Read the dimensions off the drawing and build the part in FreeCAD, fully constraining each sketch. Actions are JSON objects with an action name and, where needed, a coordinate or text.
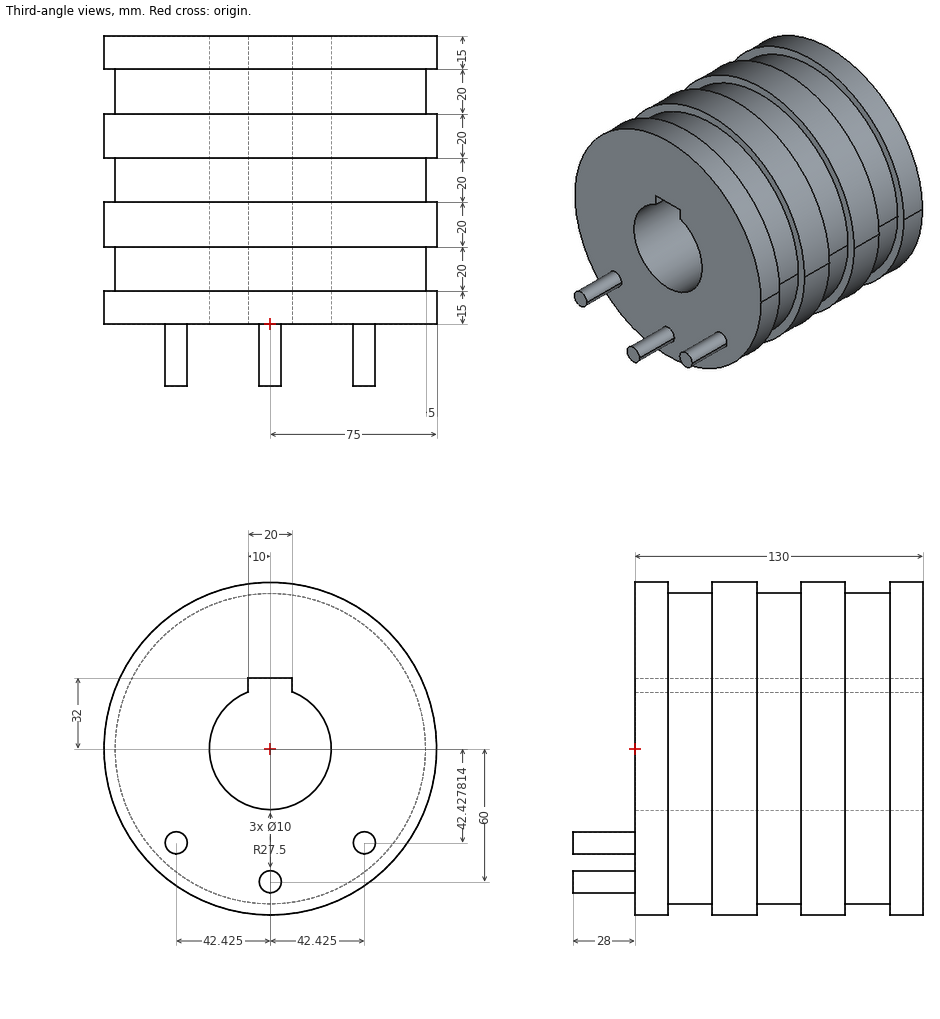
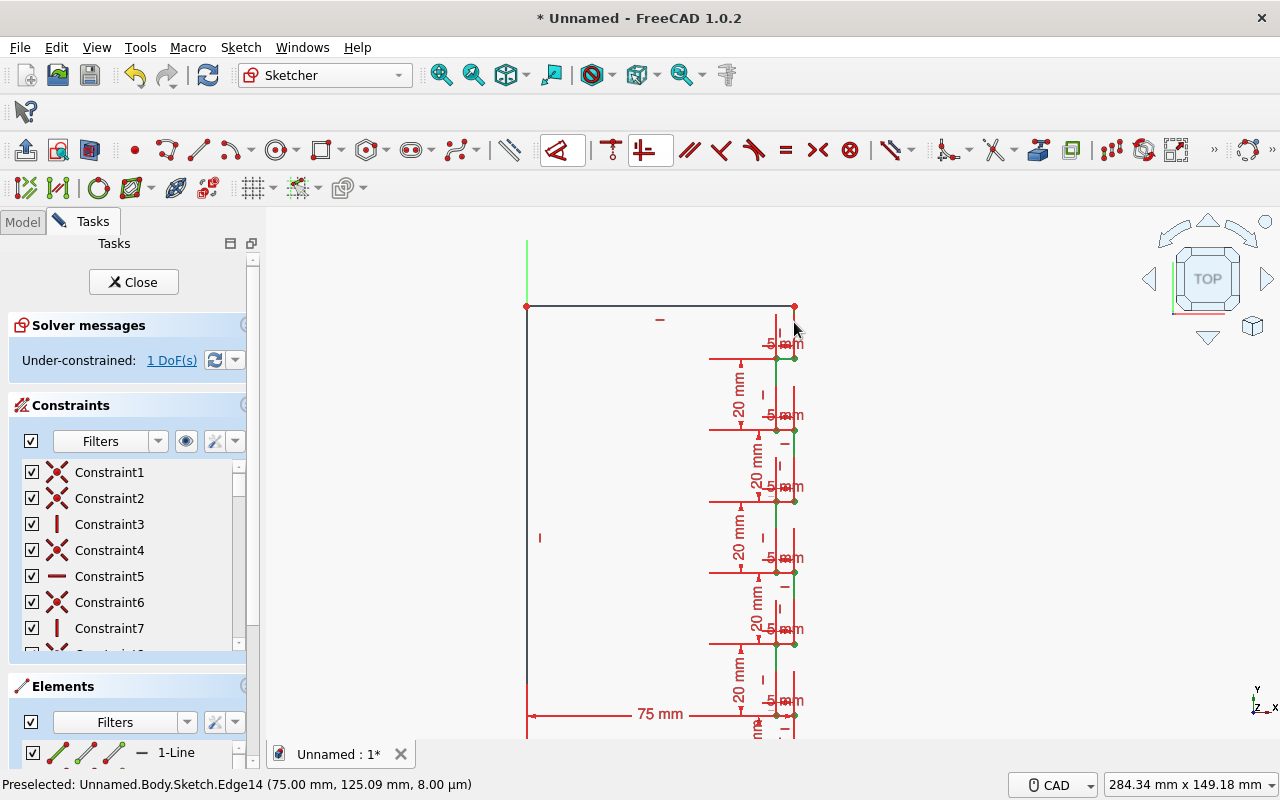
{"action": "left_click", "coordinate": [580, 150]}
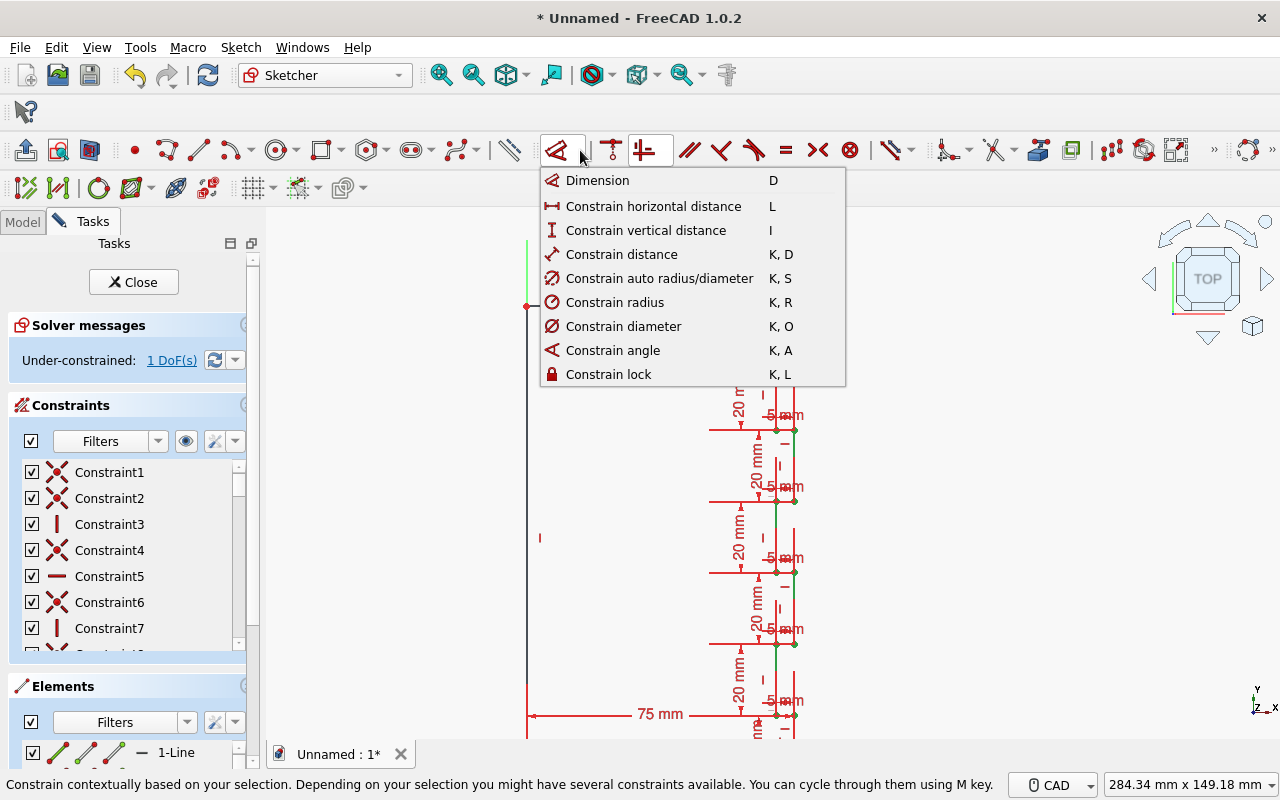
{"action": "left_click", "coordinate": [693, 230]}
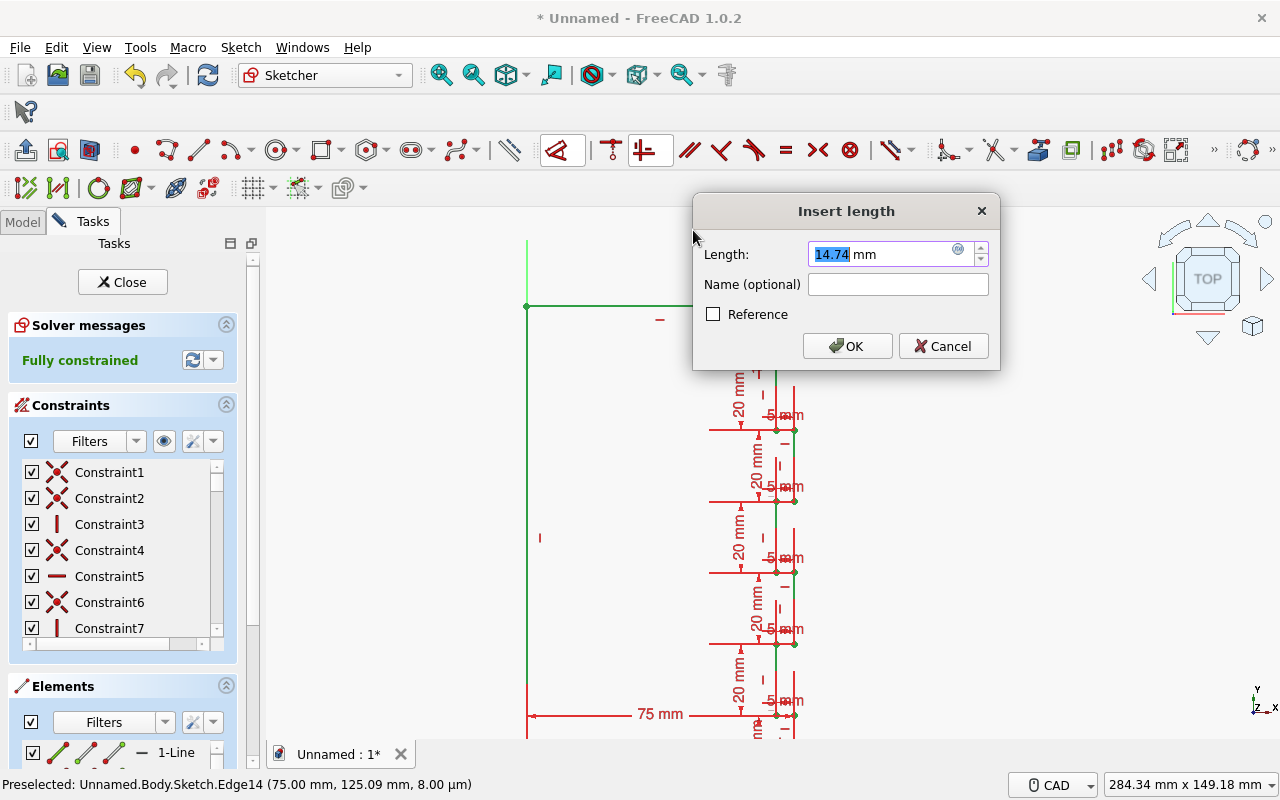
{"action": "type", "text": "15"}
{"action": "key", "text": "Return"}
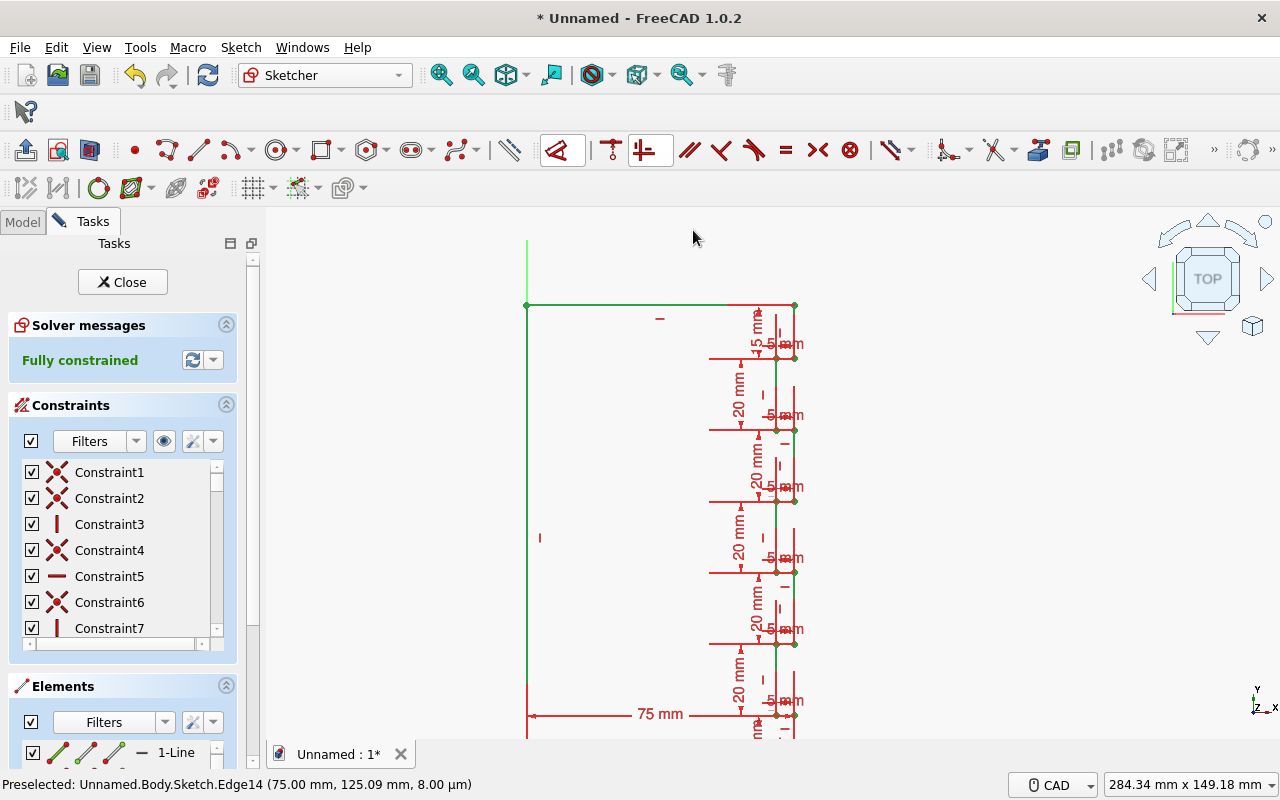
{"action": "left_click", "coordinate": [123, 282]}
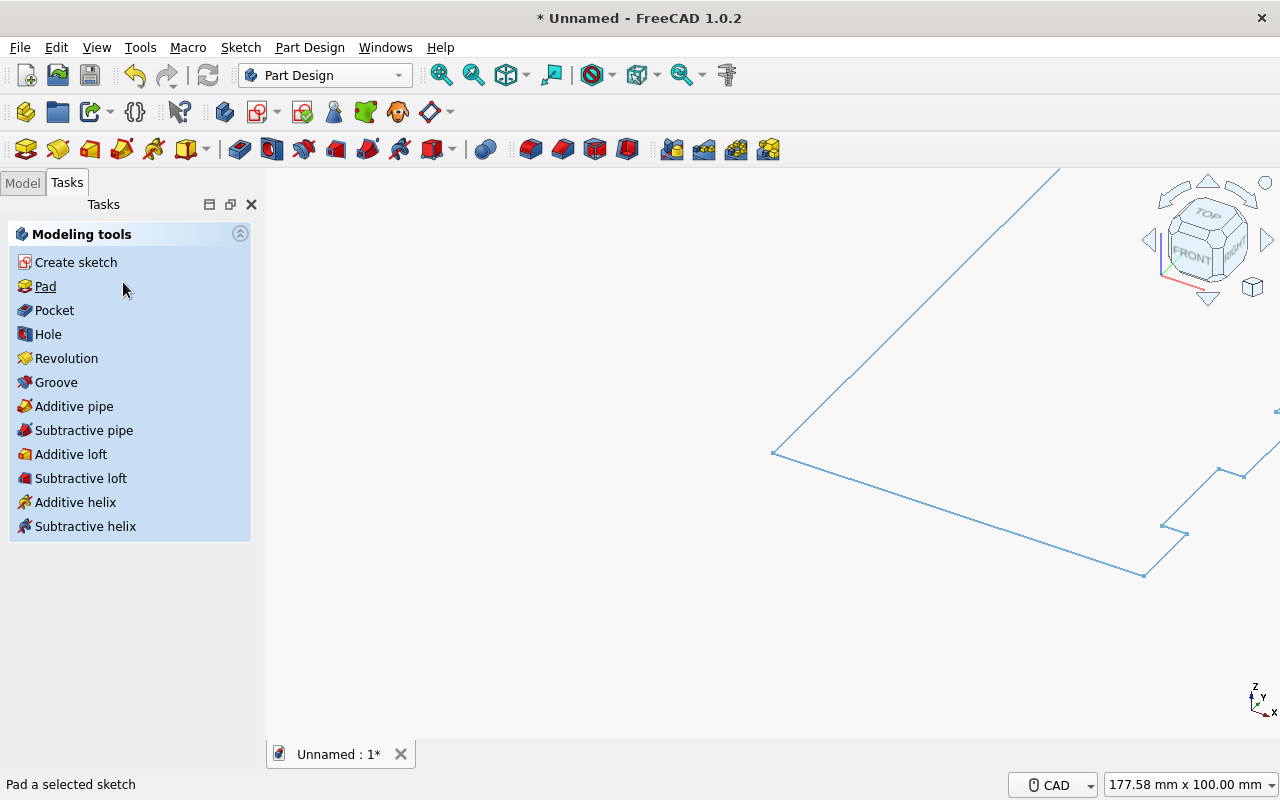
{"action": "left_click", "coordinate": [58, 150]}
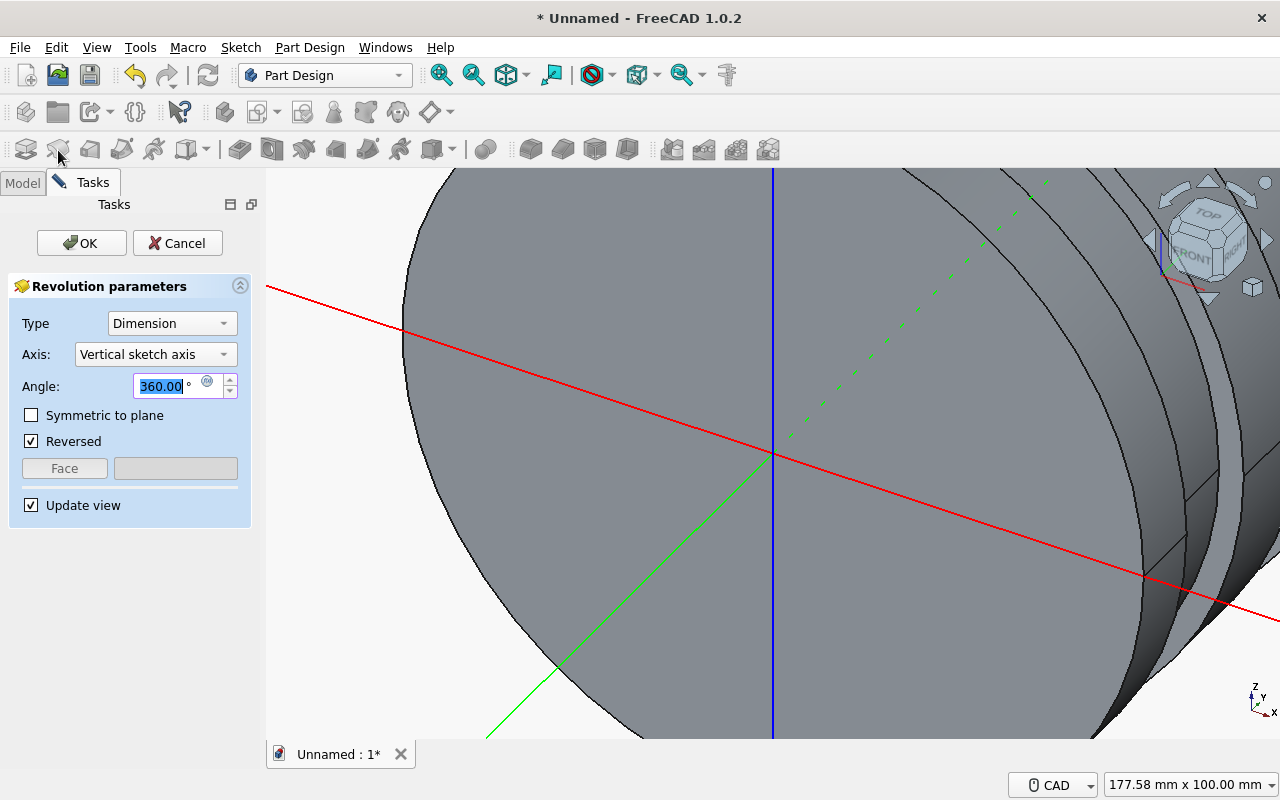
{"action": "left_click", "coordinate": [82, 243]}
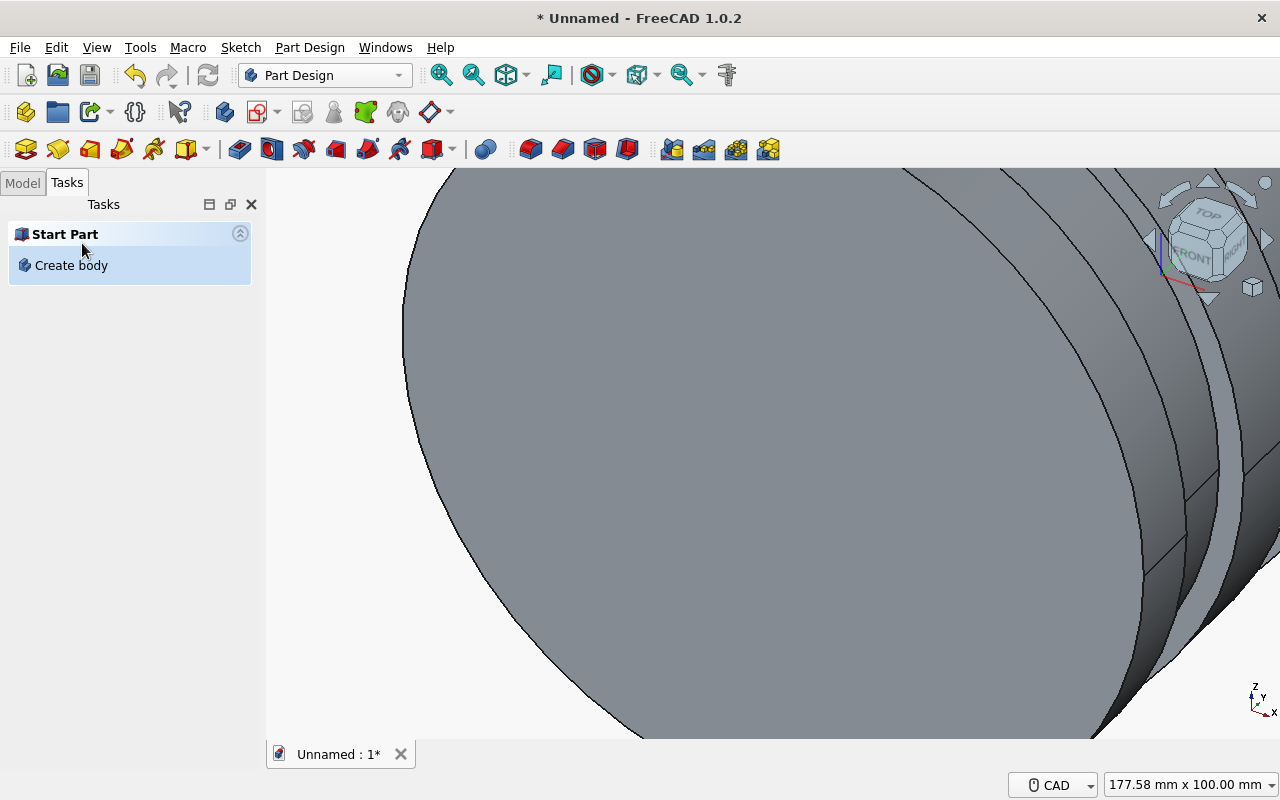
{"action": "left_click", "coordinate": [442, 76]}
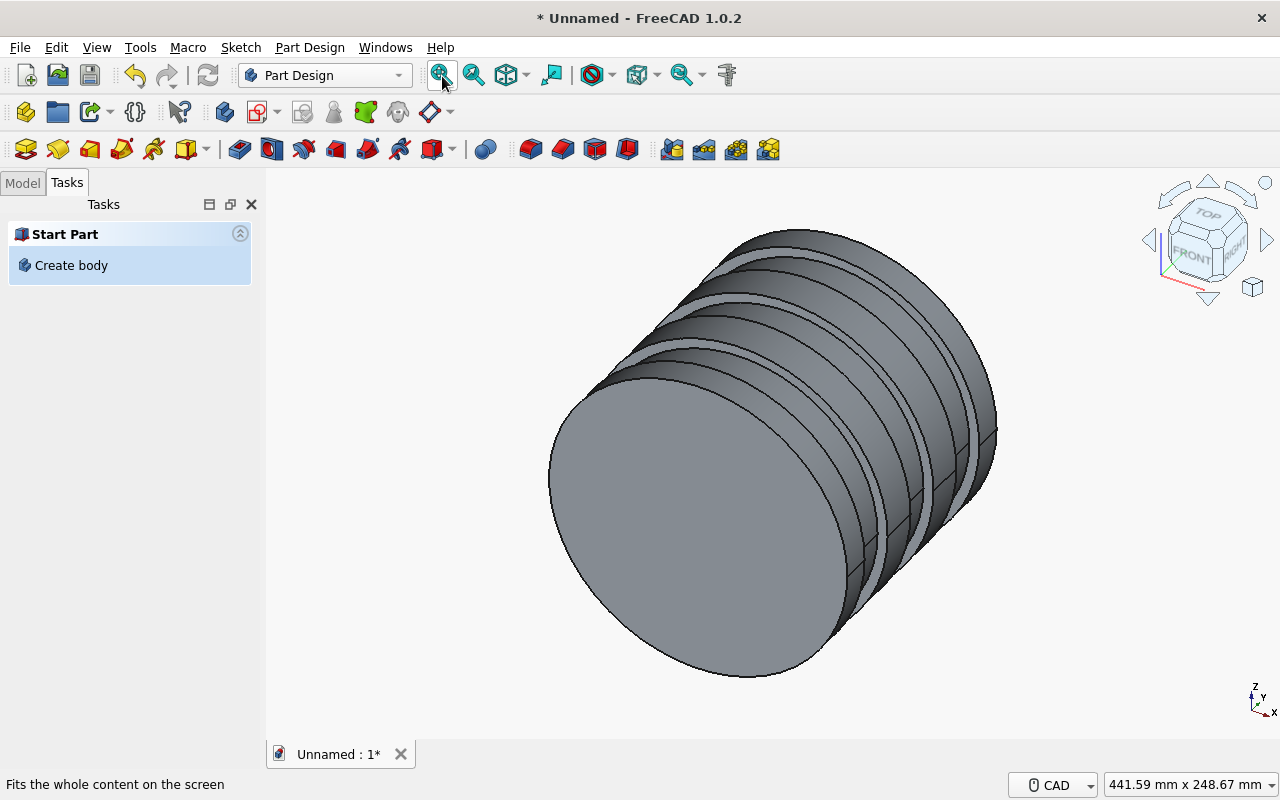
{"action": "key", "text": "4"}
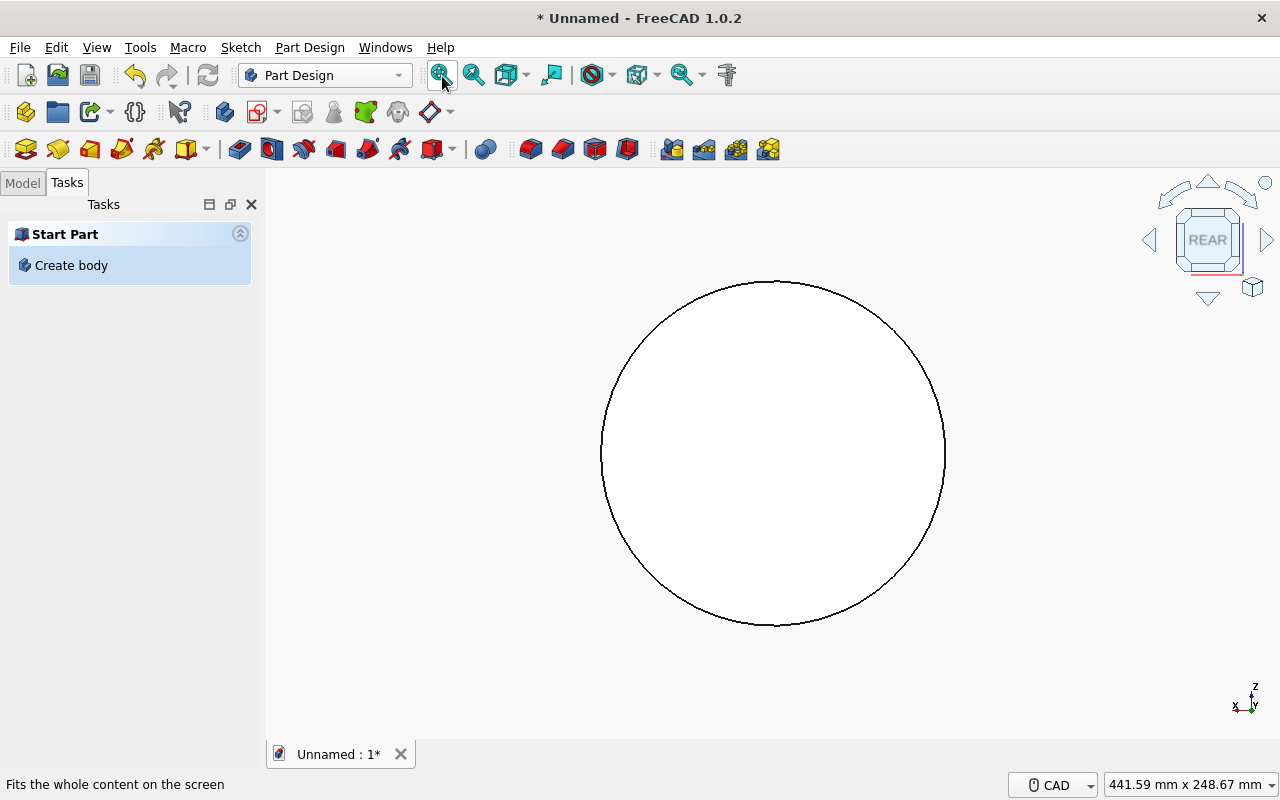
{"action": "left_click", "coordinate": [773, 453]}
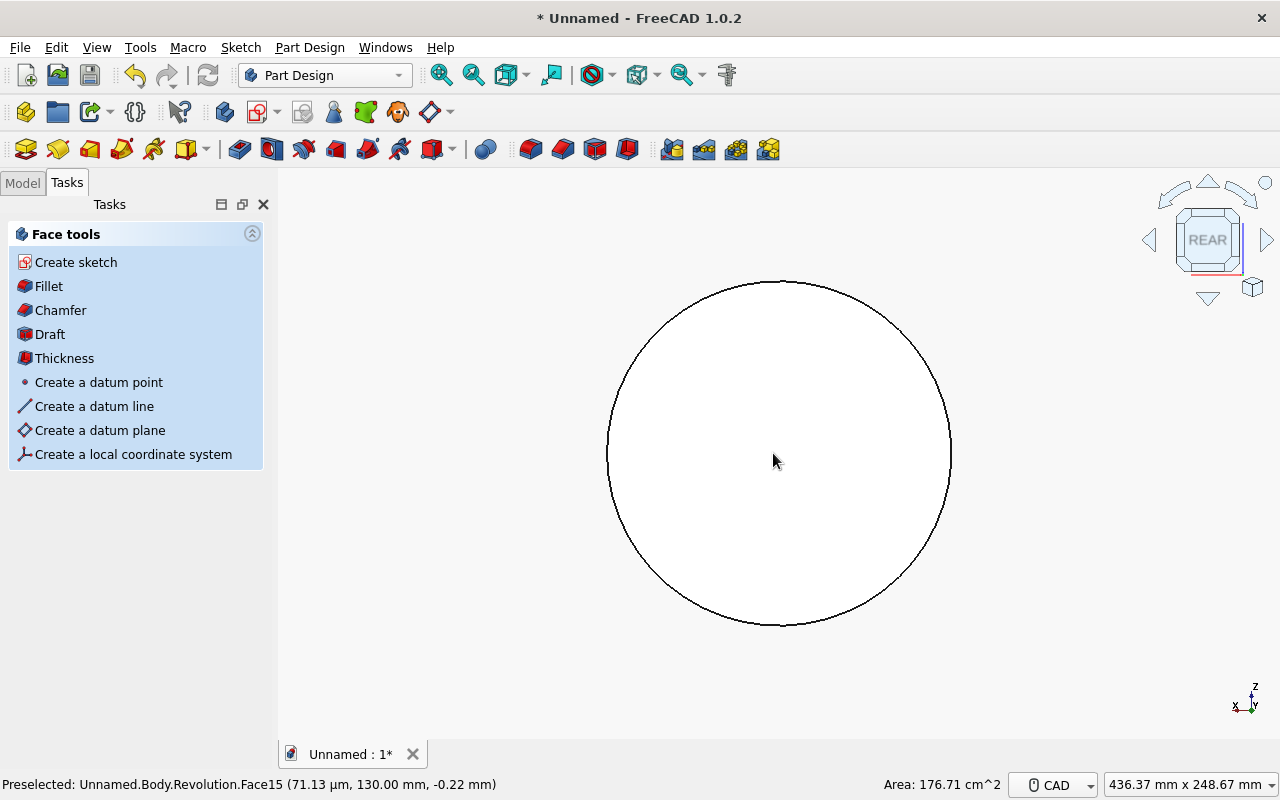
{"action": "left_click", "coordinate": [258, 112]}